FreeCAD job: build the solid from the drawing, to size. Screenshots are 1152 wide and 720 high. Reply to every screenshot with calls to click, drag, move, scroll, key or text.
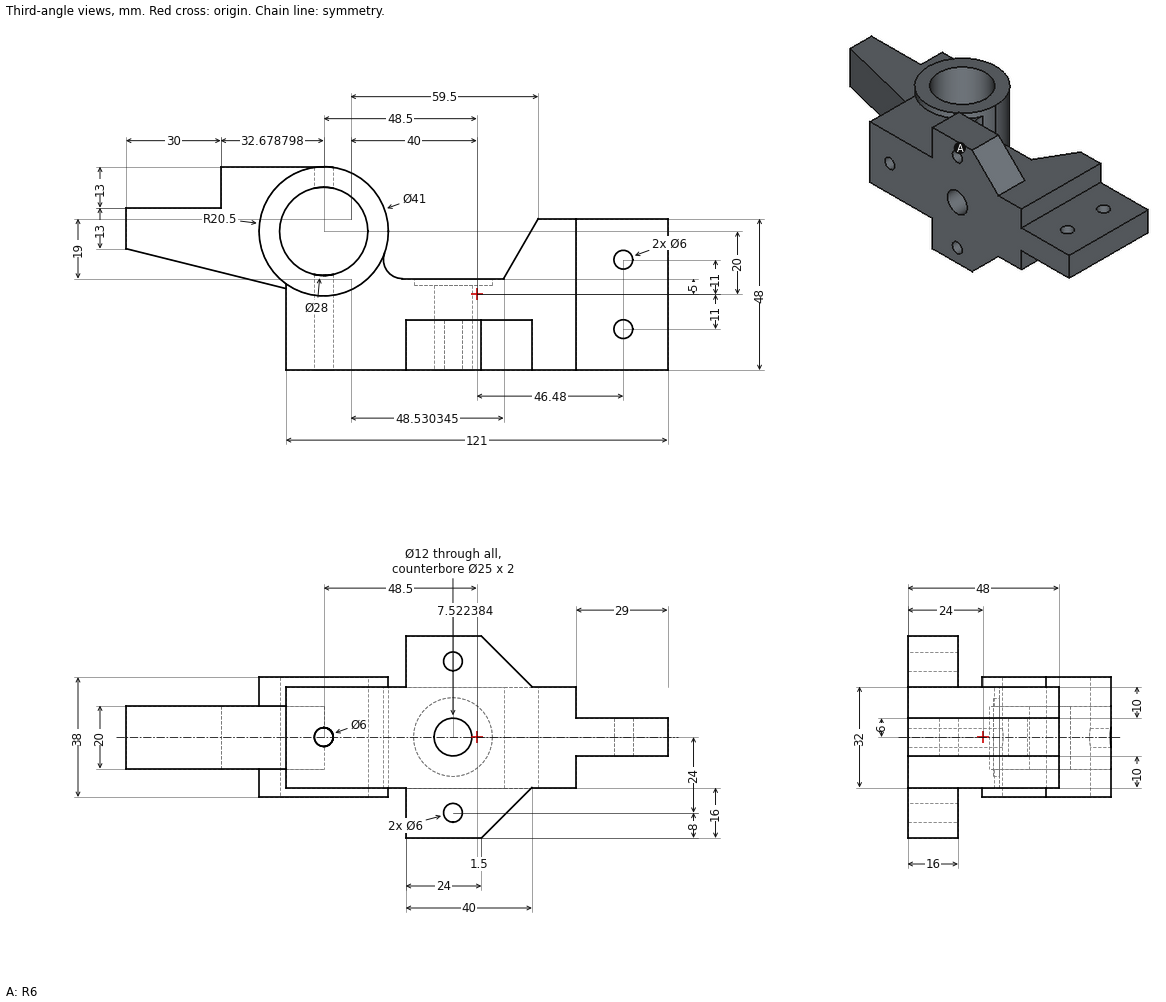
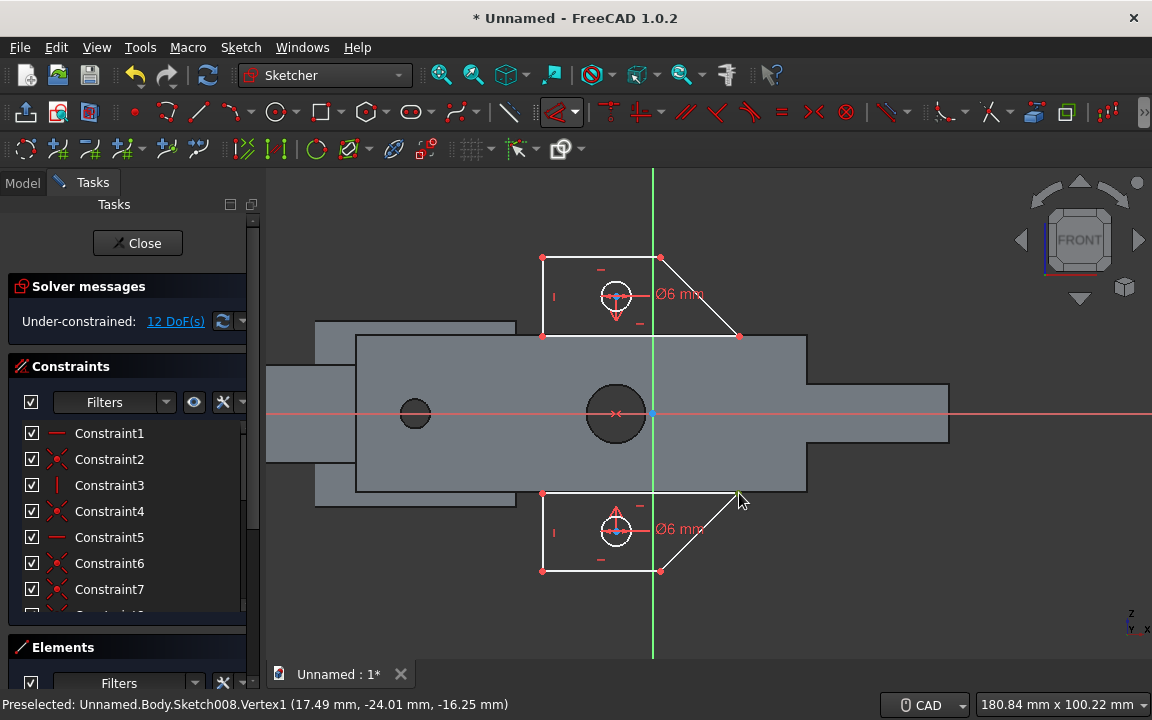
click(739, 336)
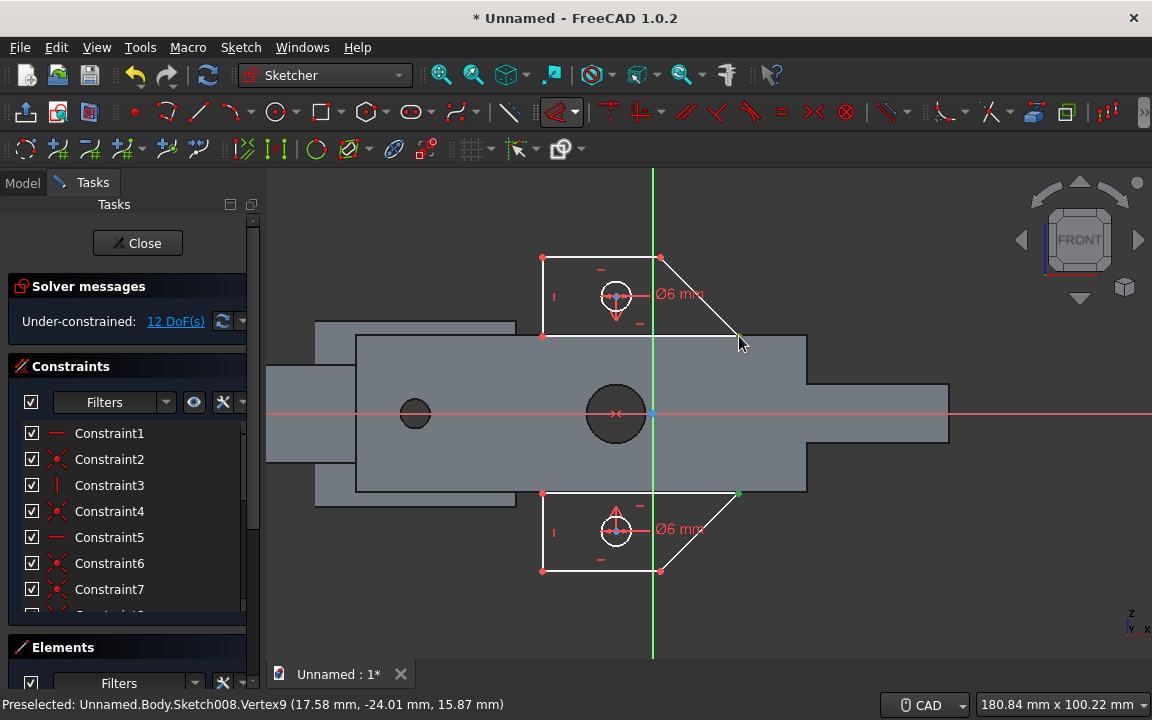
click(344, 414)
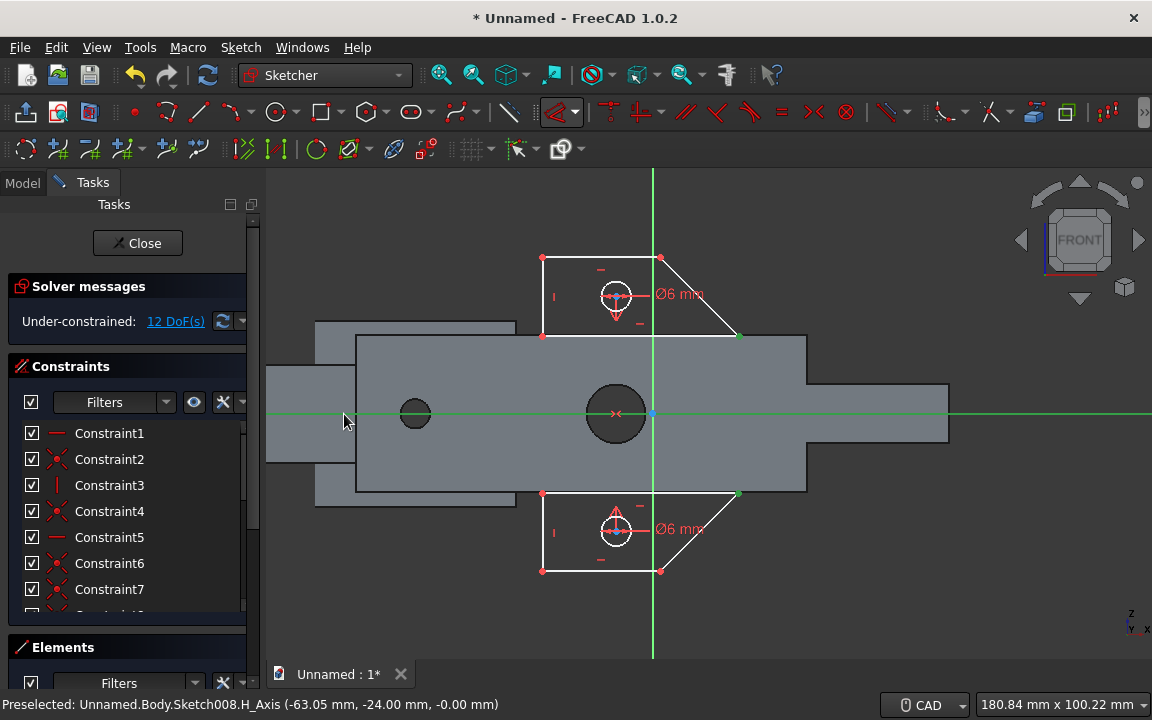
click(814, 112)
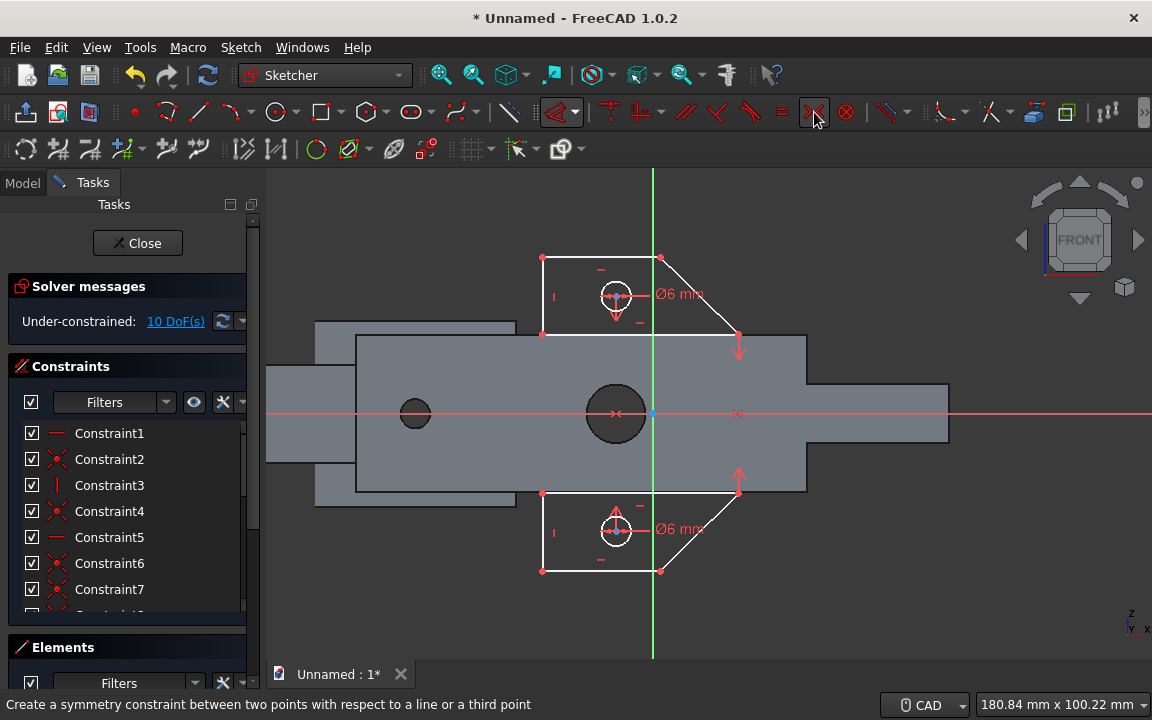
click(660, 571)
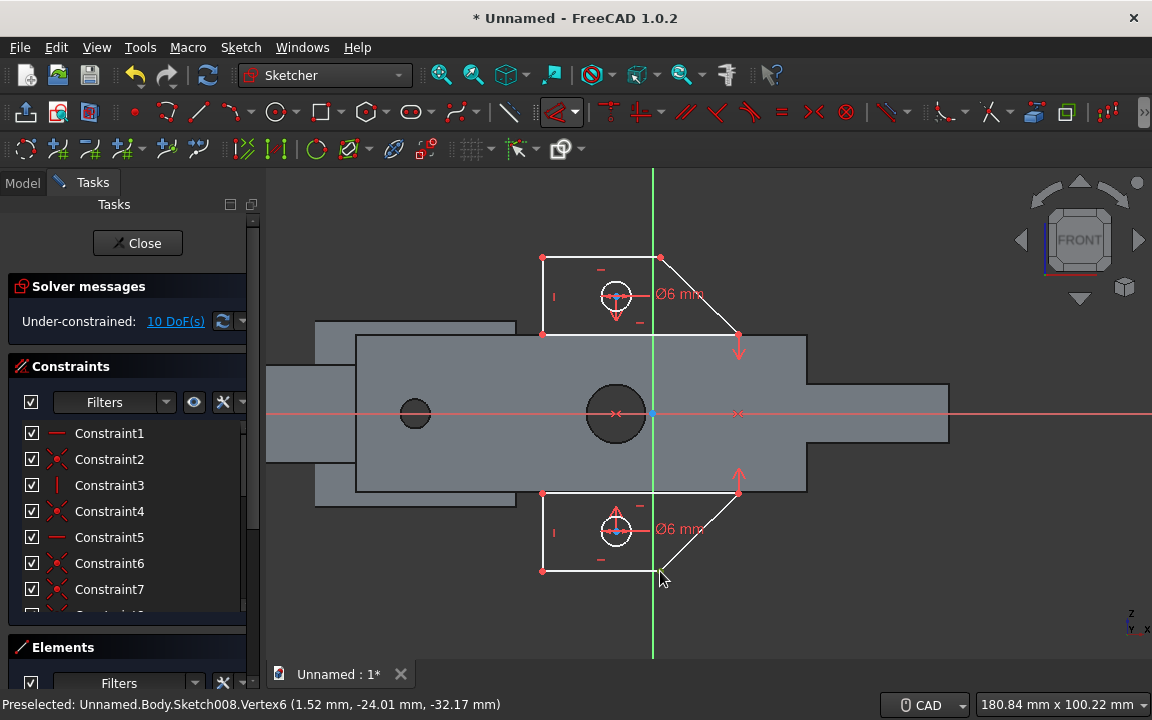
click(660, 257)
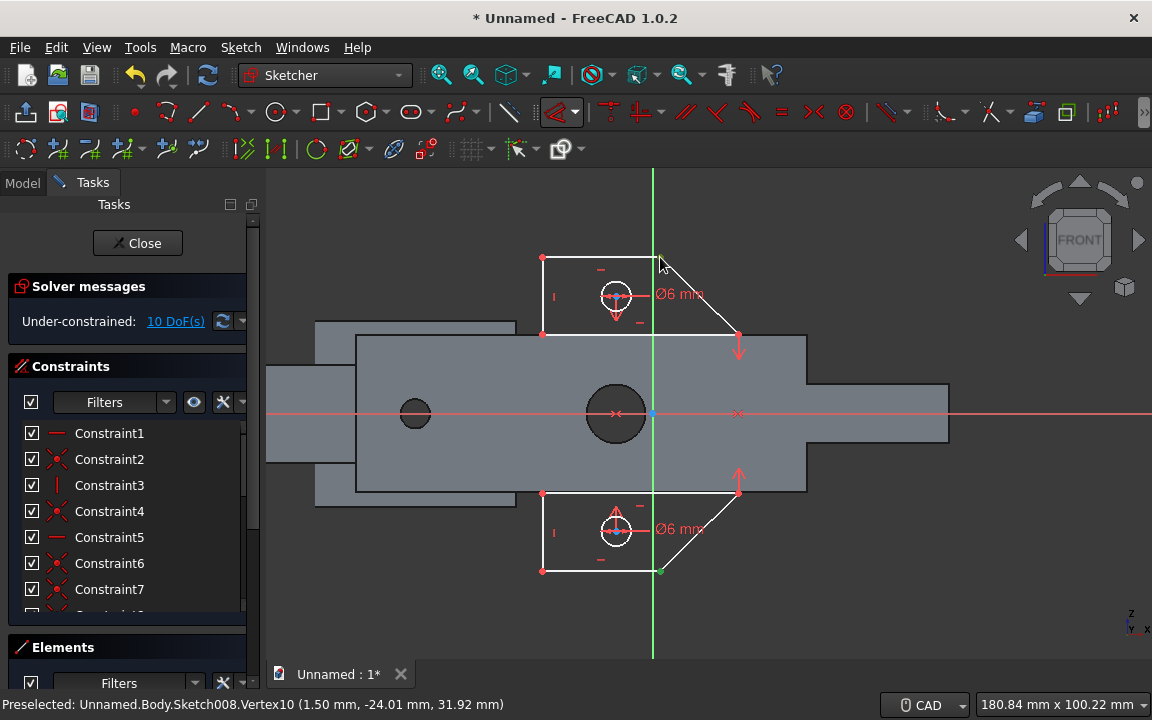
click(344, 414)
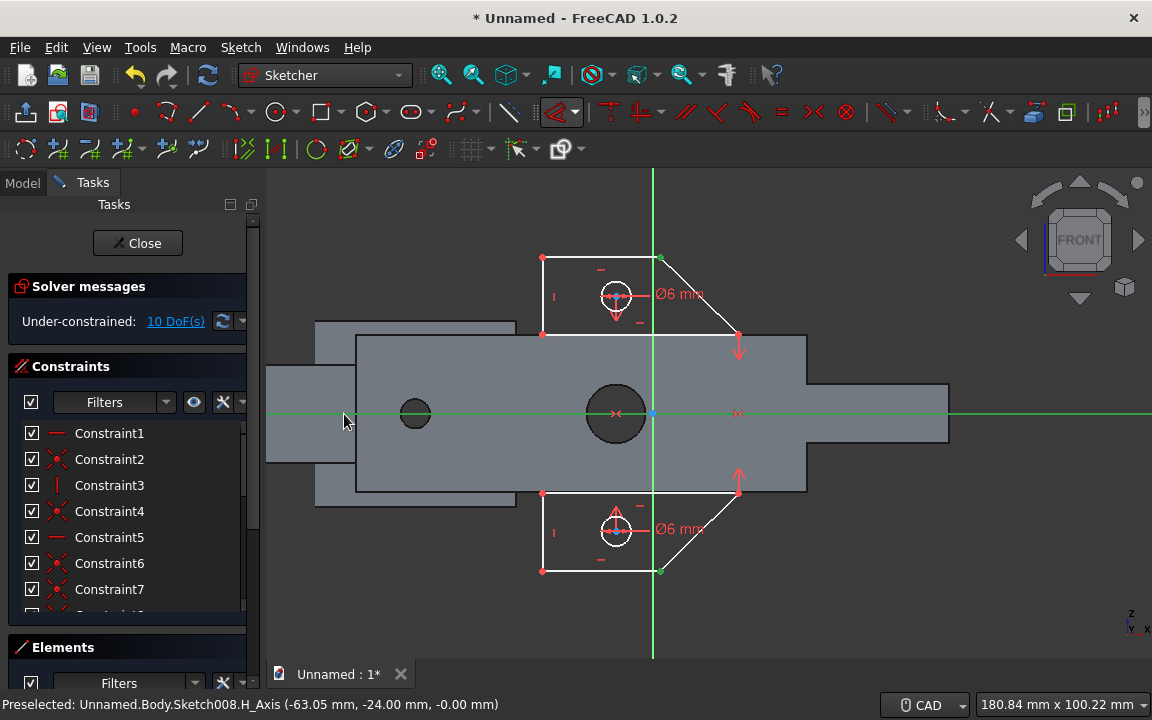
key(s)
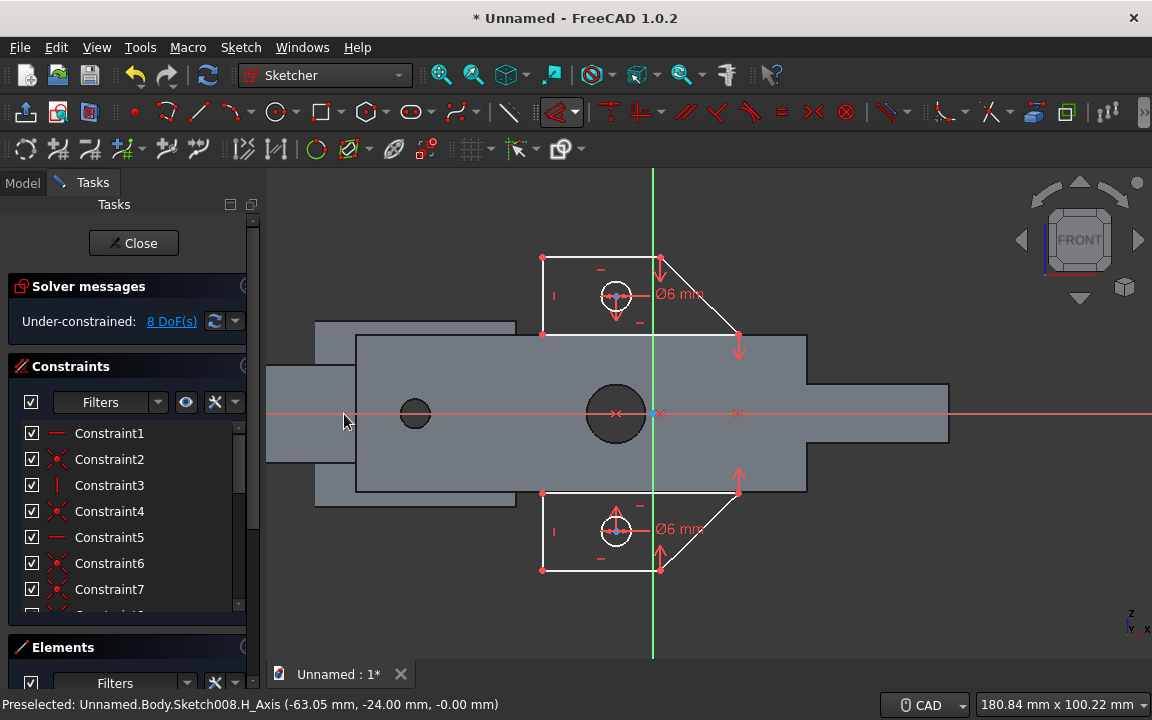
click(680, 493)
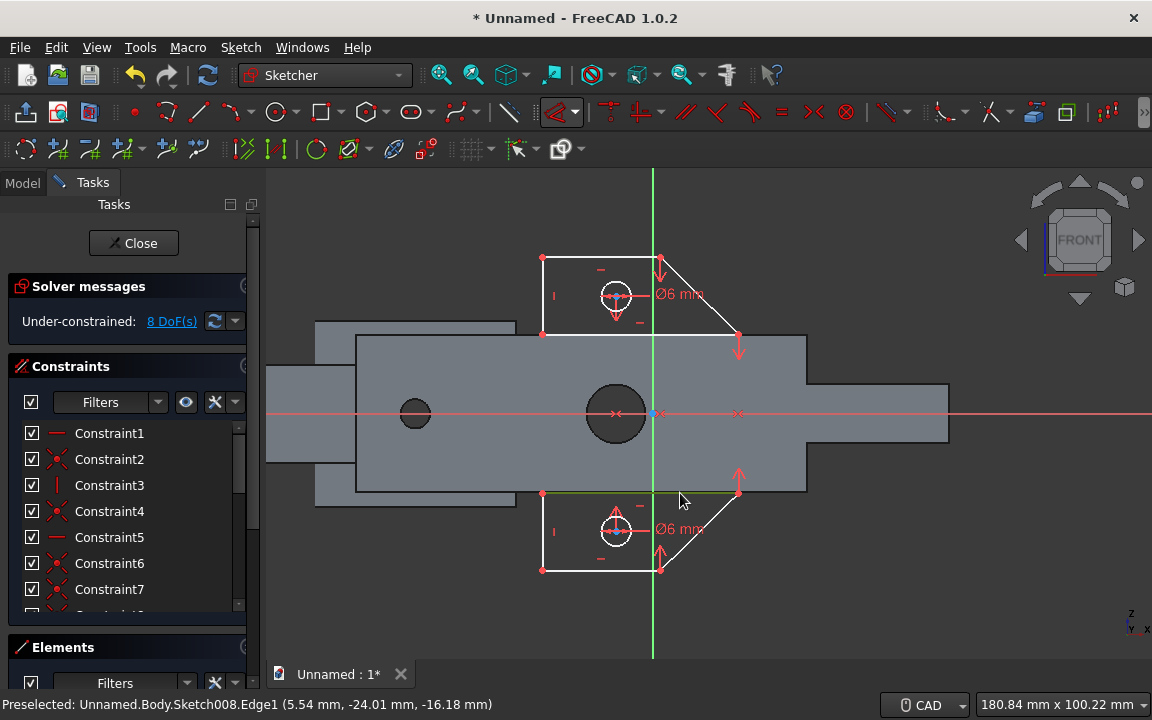
key(l)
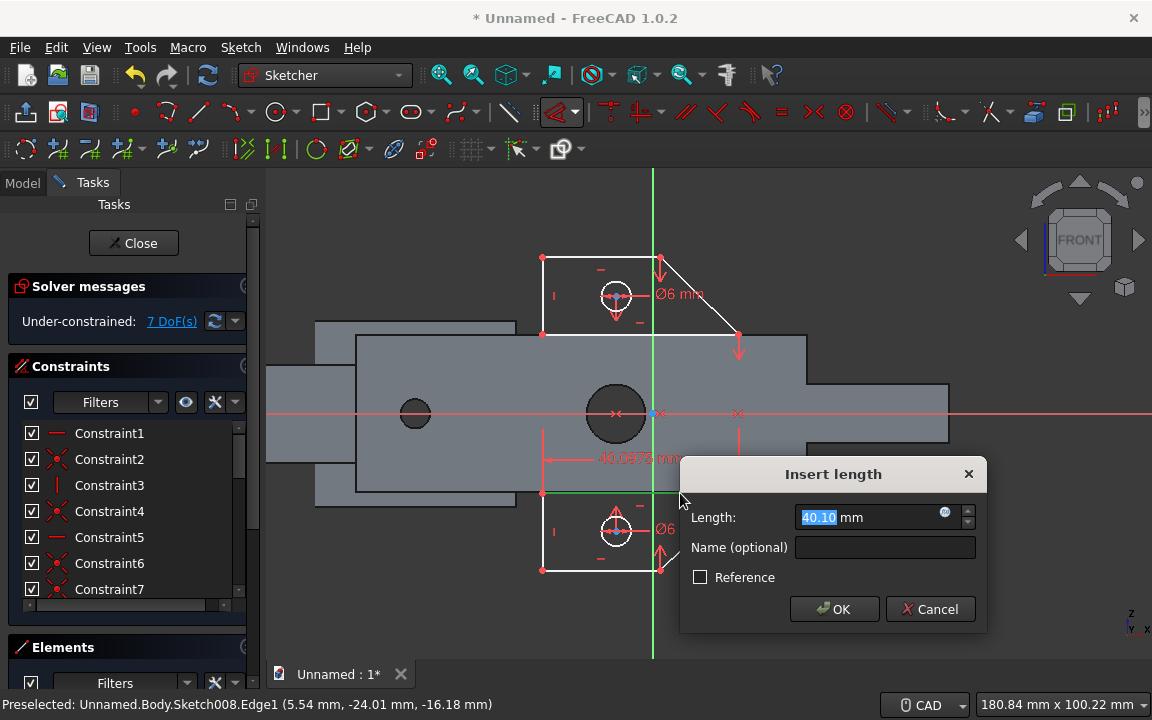
text(40)
key(Return)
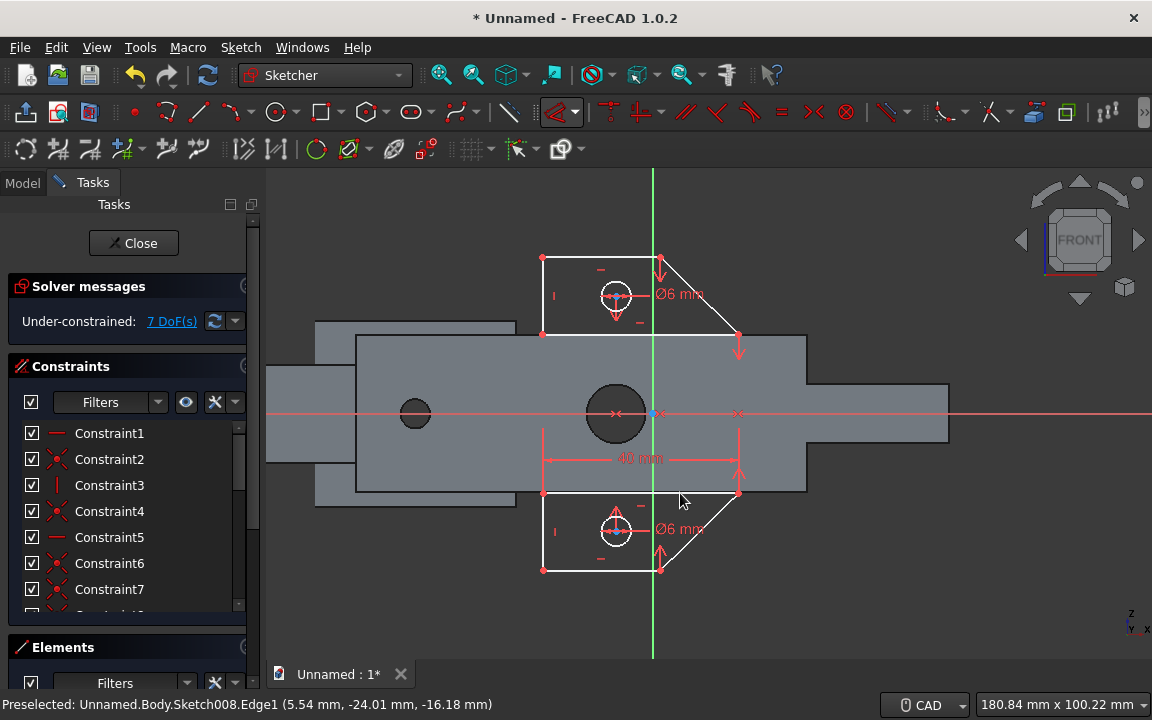
click(543, 516)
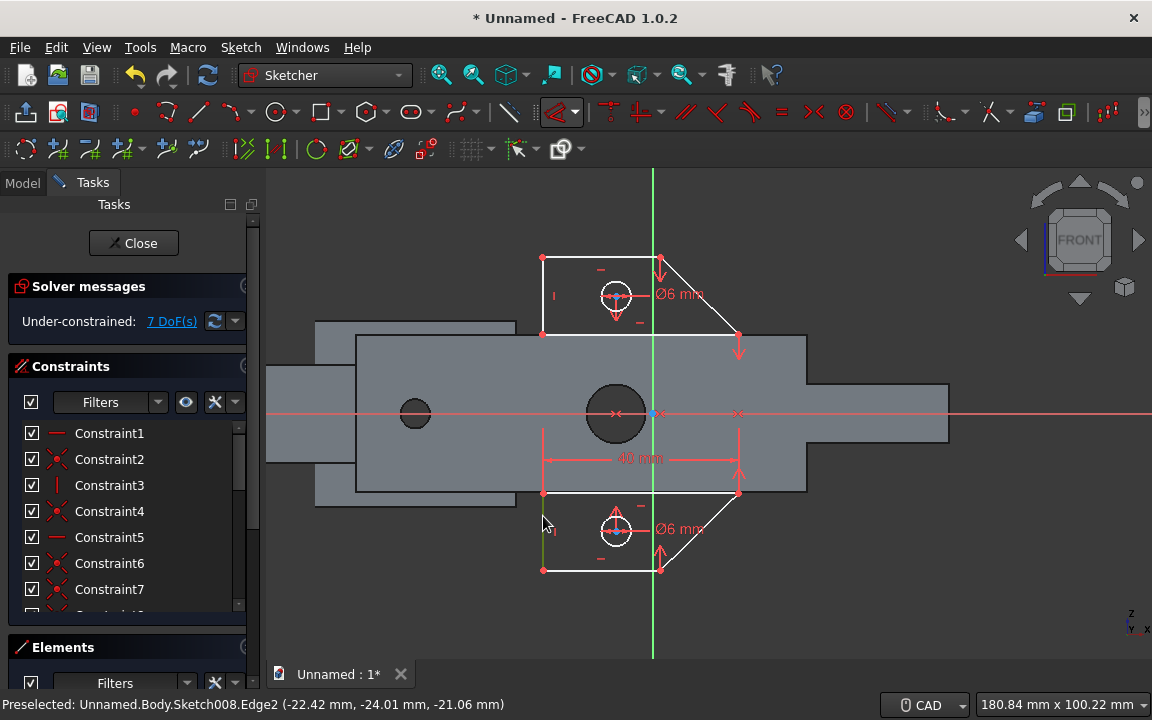
key(i)